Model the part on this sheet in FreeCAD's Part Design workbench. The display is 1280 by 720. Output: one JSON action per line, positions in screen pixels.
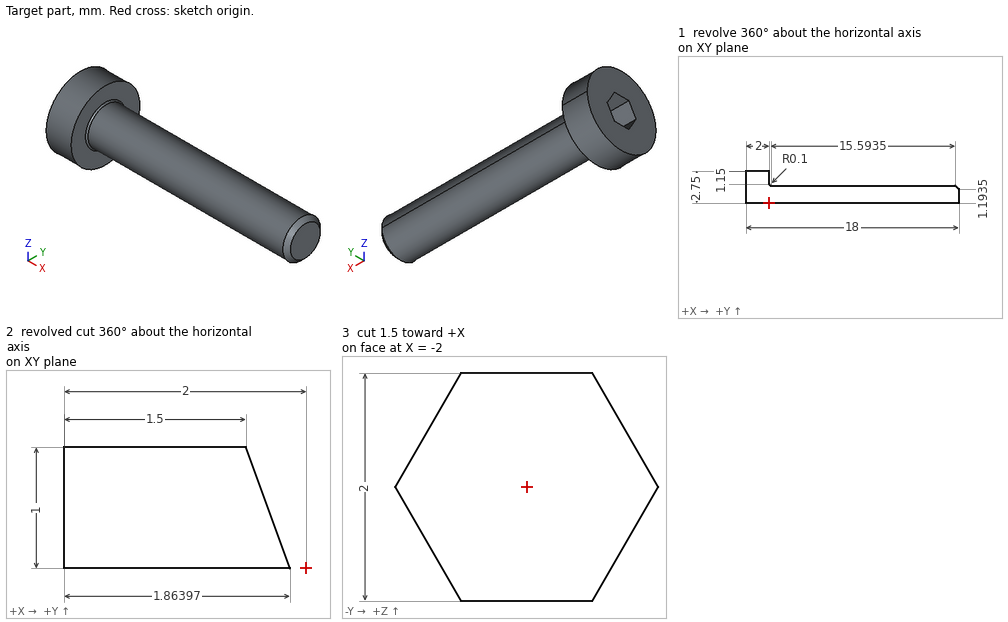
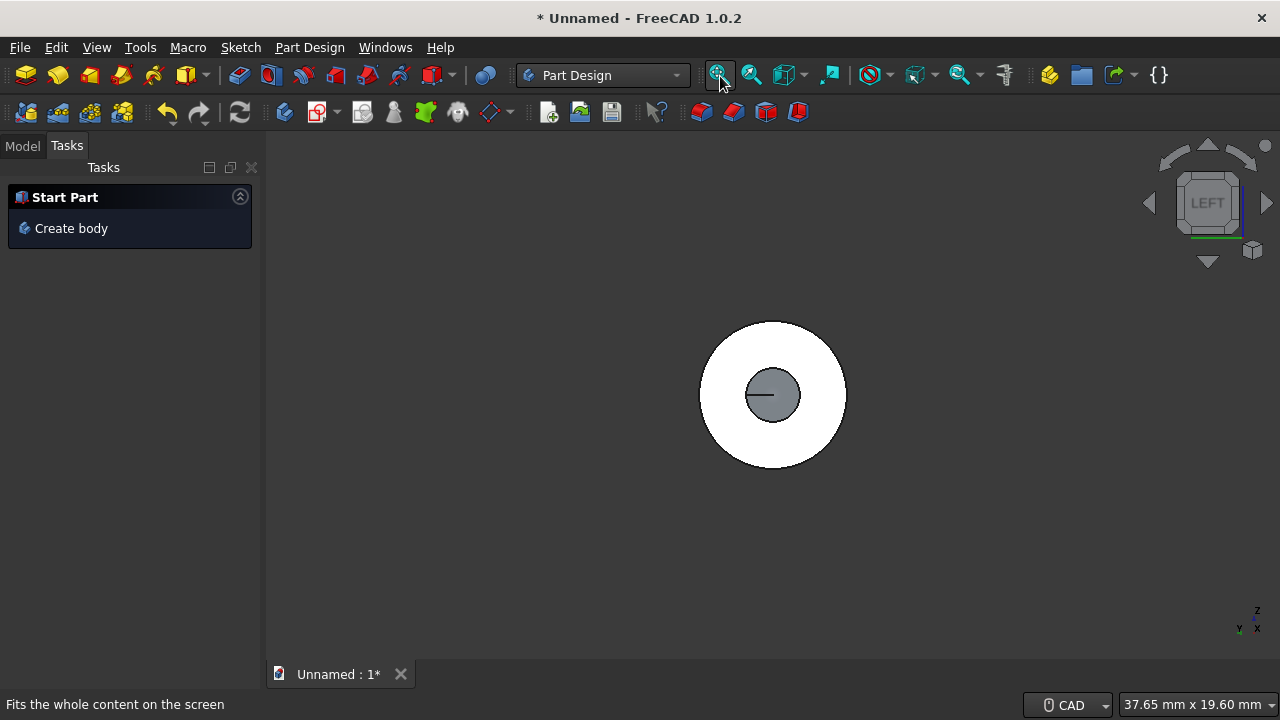
{"action": "left_click", "coordinate": [794, 436]}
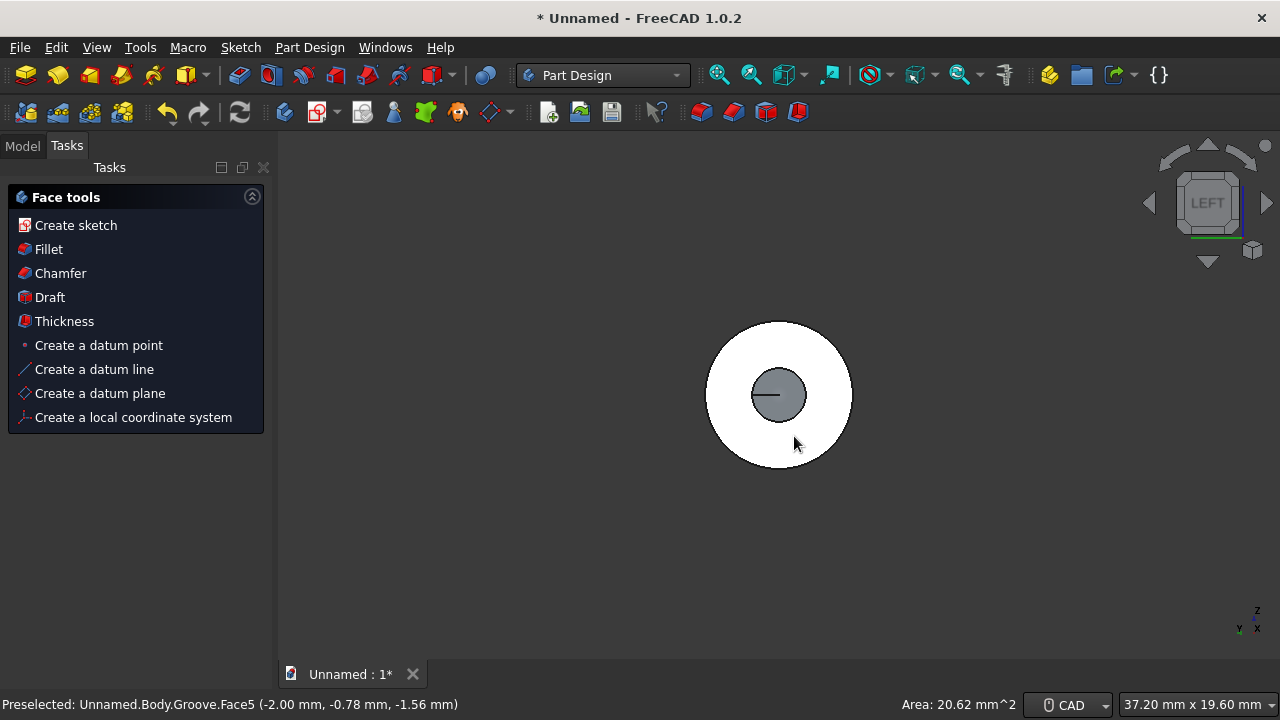
{"action": "left_click", "coordinate": [318, 112]}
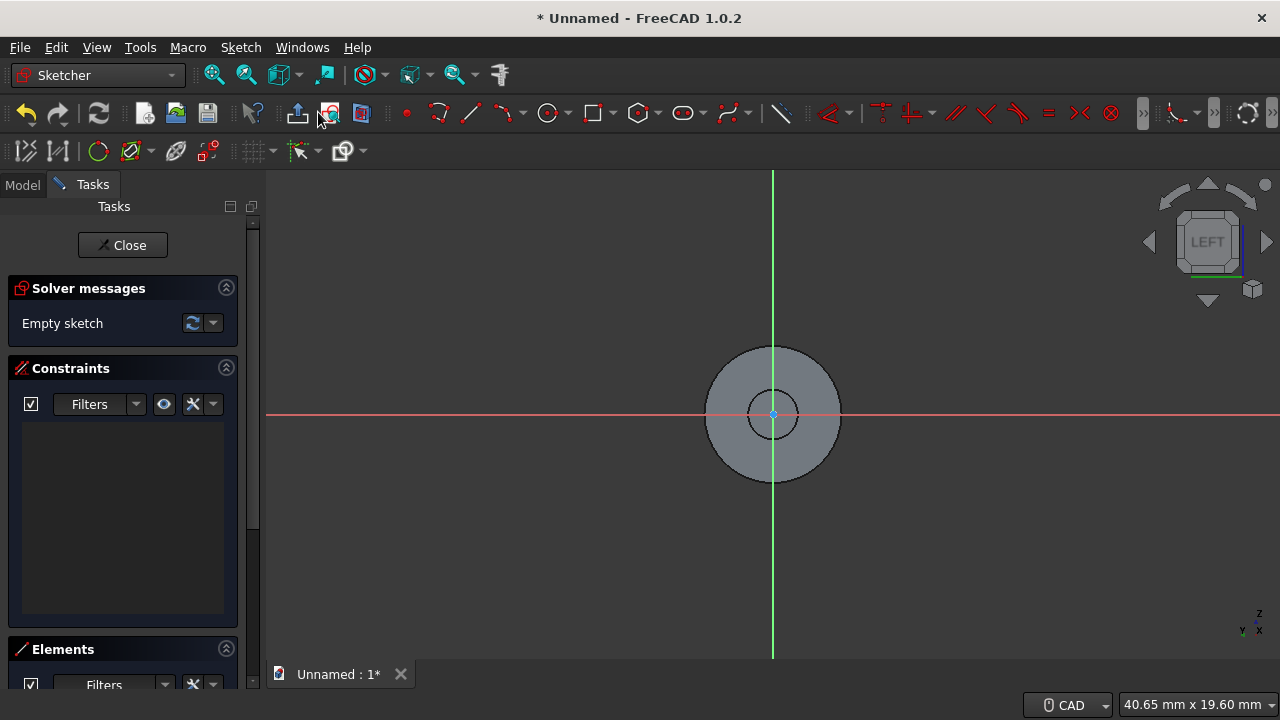
{"action": "scroll", "coordinate": [787, 414], "scroll_direction": "up", "scroll_amount": 9}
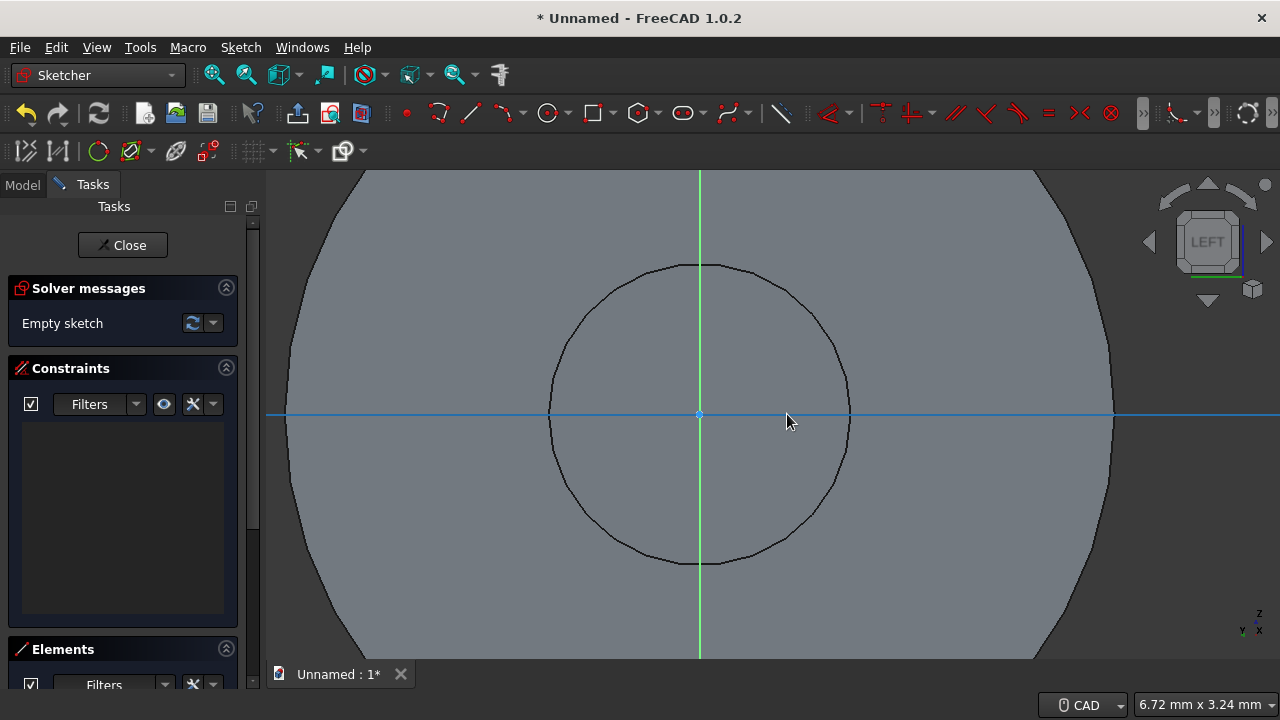
{"action": "left_click", "coordinate": [638, 114]}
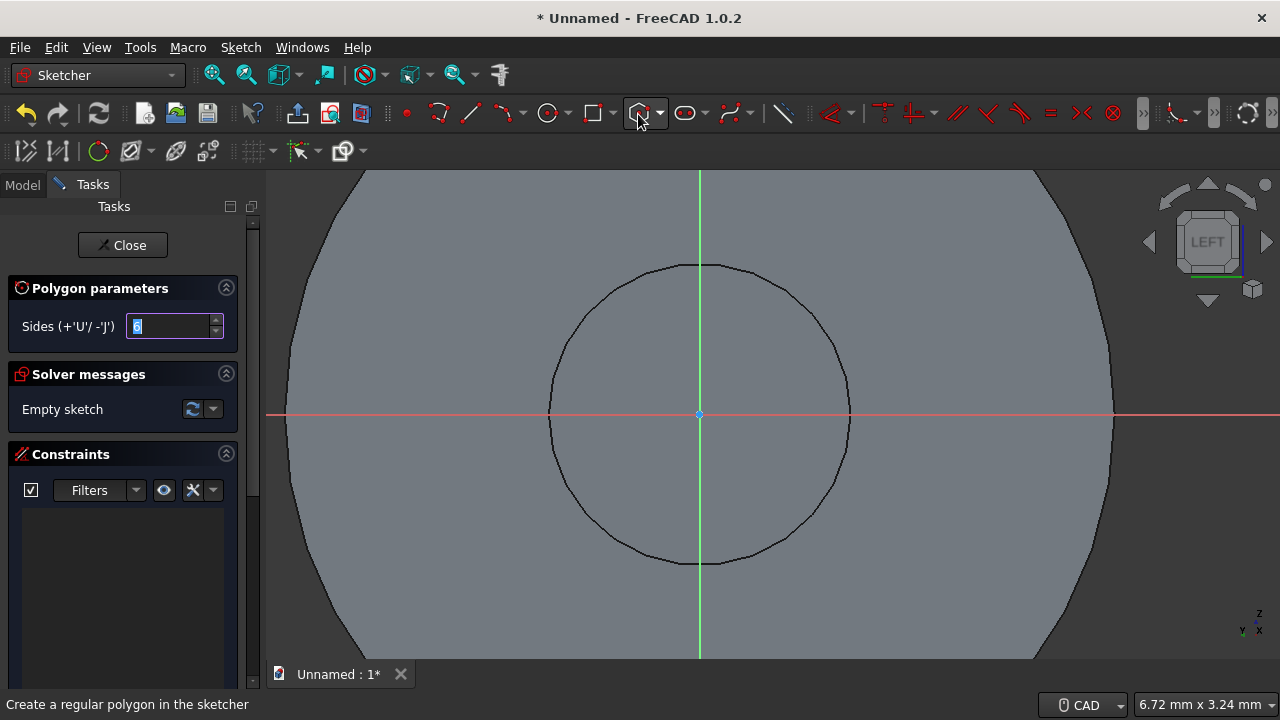
{"action": "left_click", "coordinate": [700, 414]}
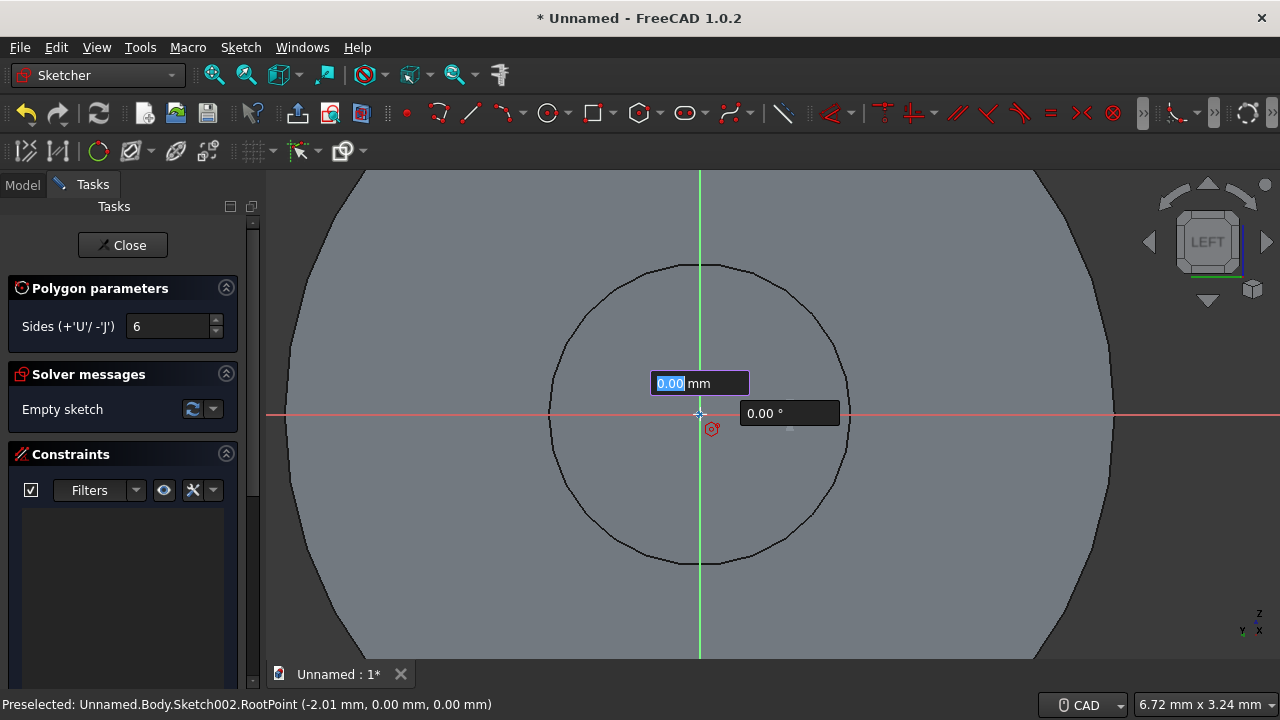
{"action": "left_click", "coordinate": [874, 414]}
{"action": "key", "text": "Escape"}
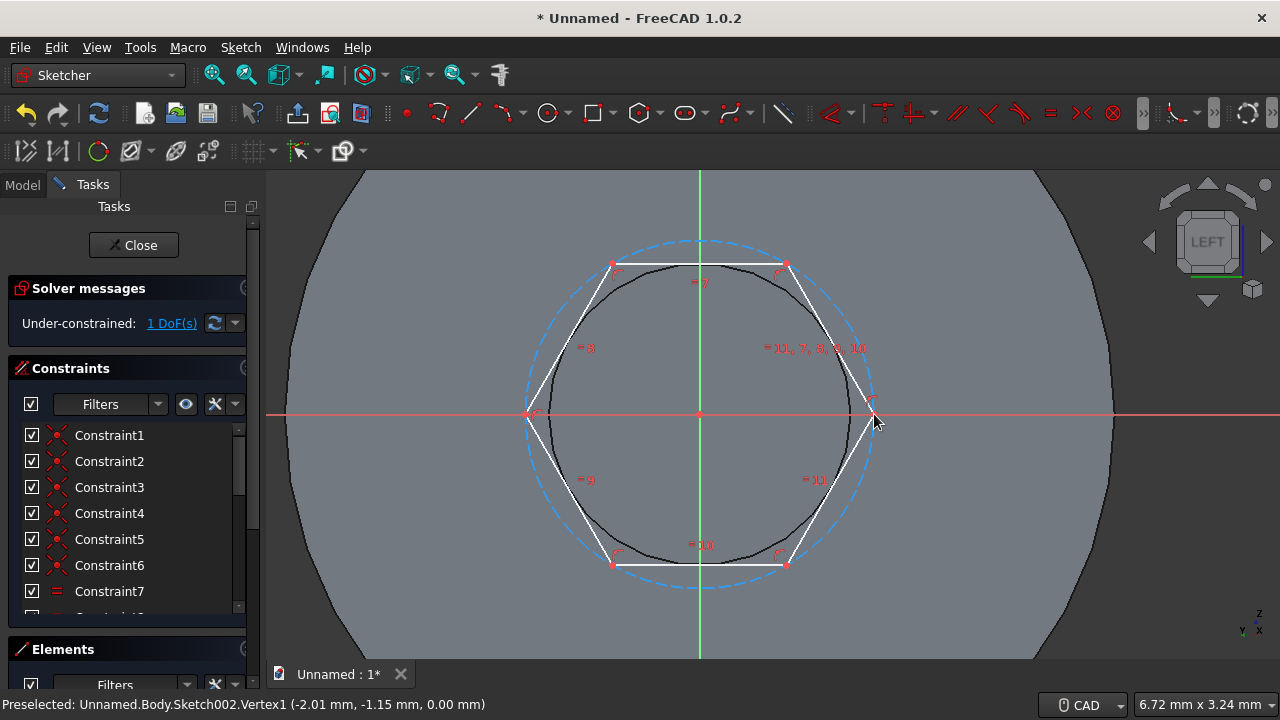
{"action": "left_click", "coordinate": [830, 114]}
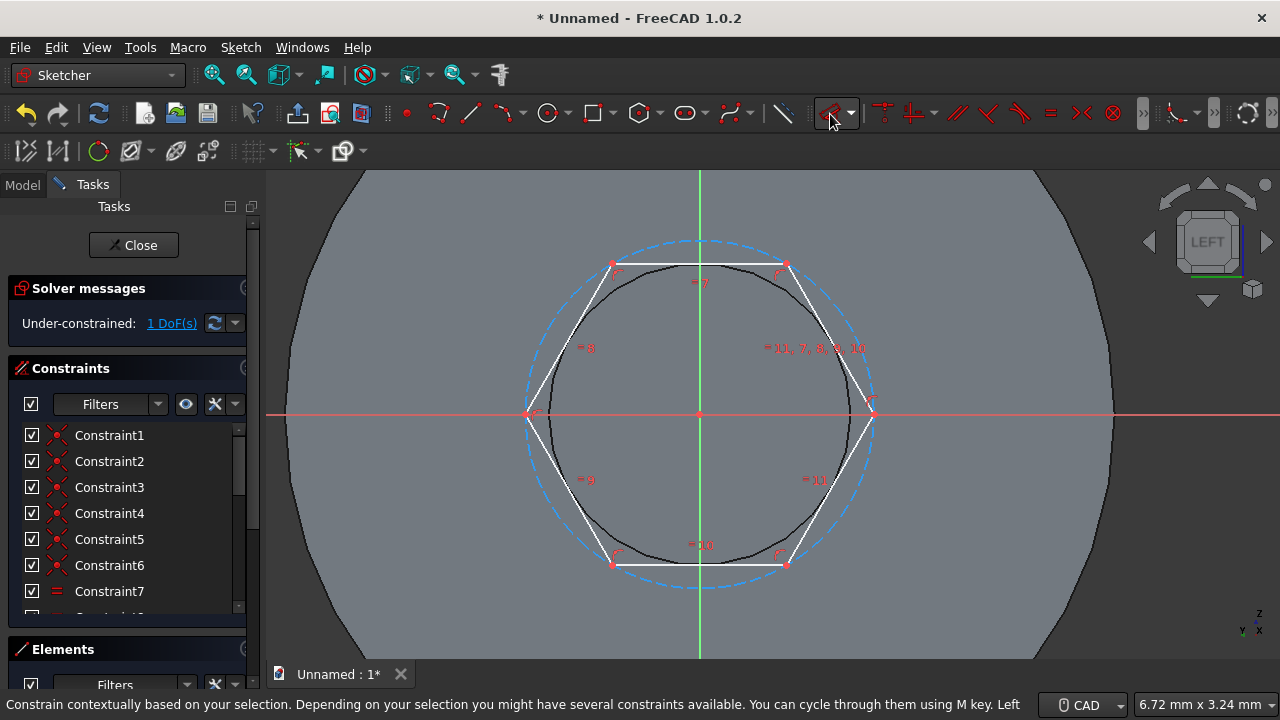
{"action": "left_click", "coordinate": [613, 565]}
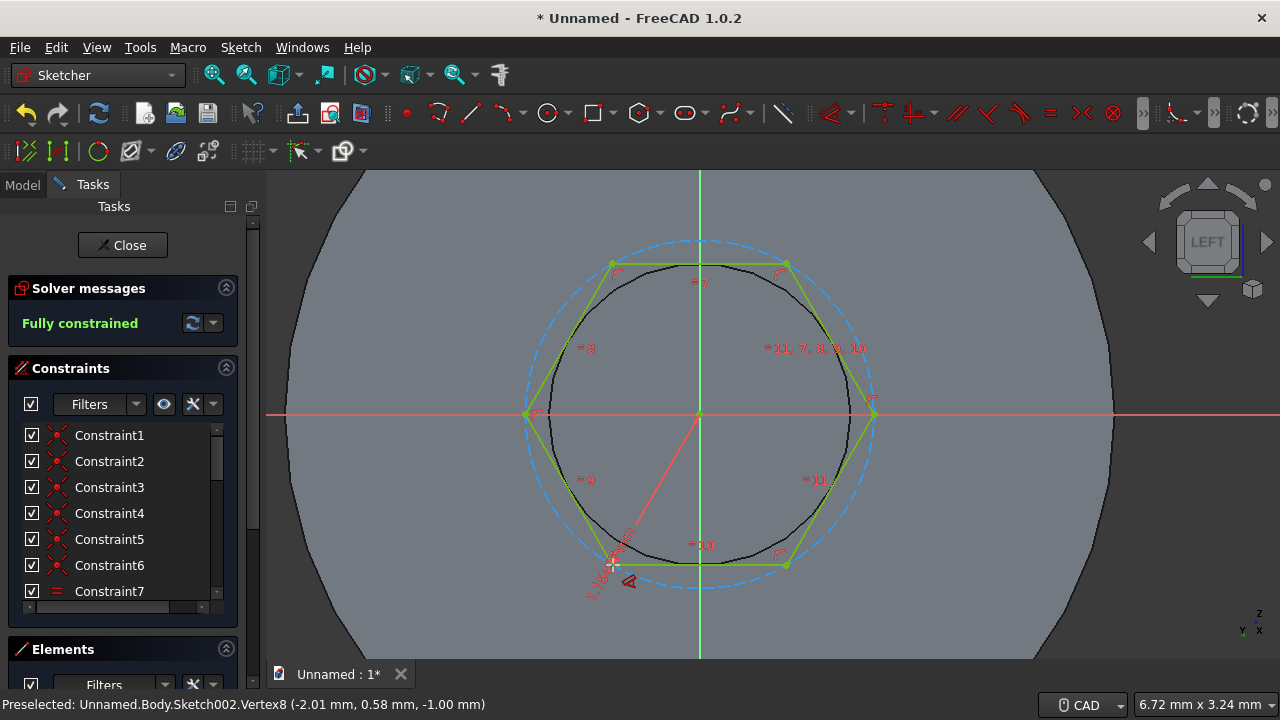
{"action": "left_click", "coordinate": [787, 264]}
{"action": "left_click", "coordinate": [869, 309]}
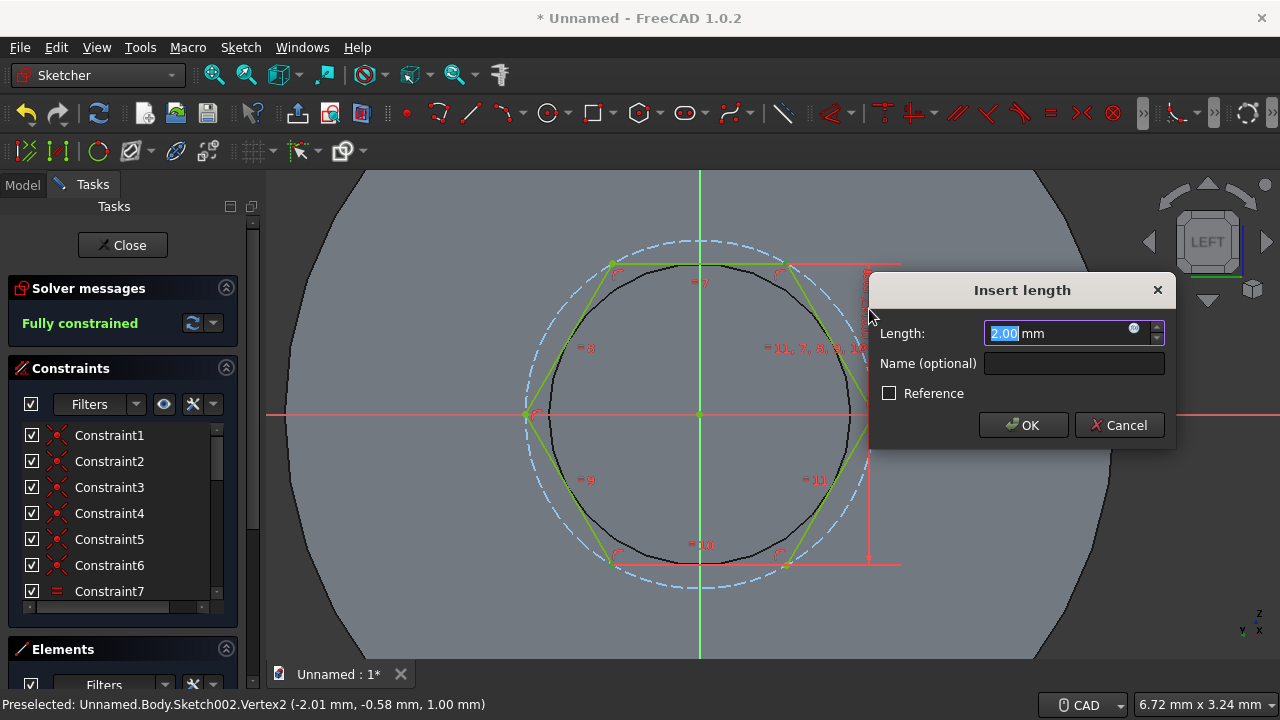
{"action": "type", "text": "2"}
{"action": "key", "text": "Return"}
{"action": "key", "text": "Escape"}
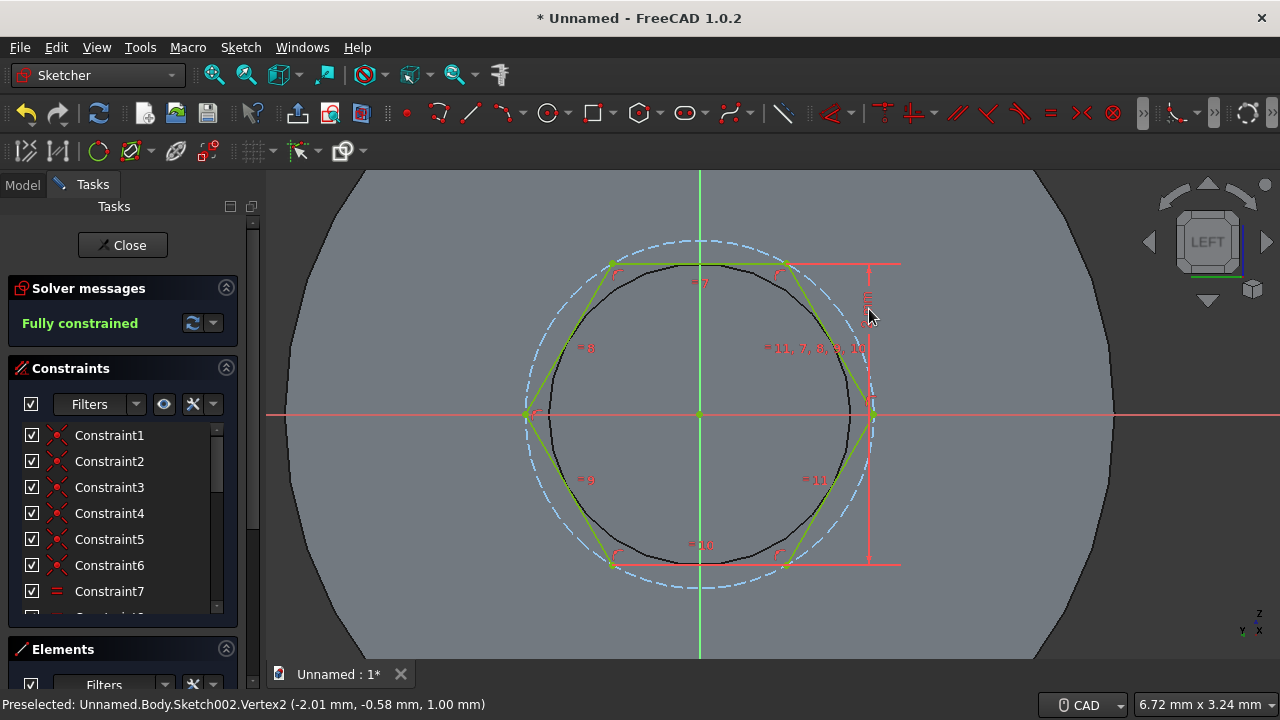
{"action": "left_click", "coordinate": [123, 245]}